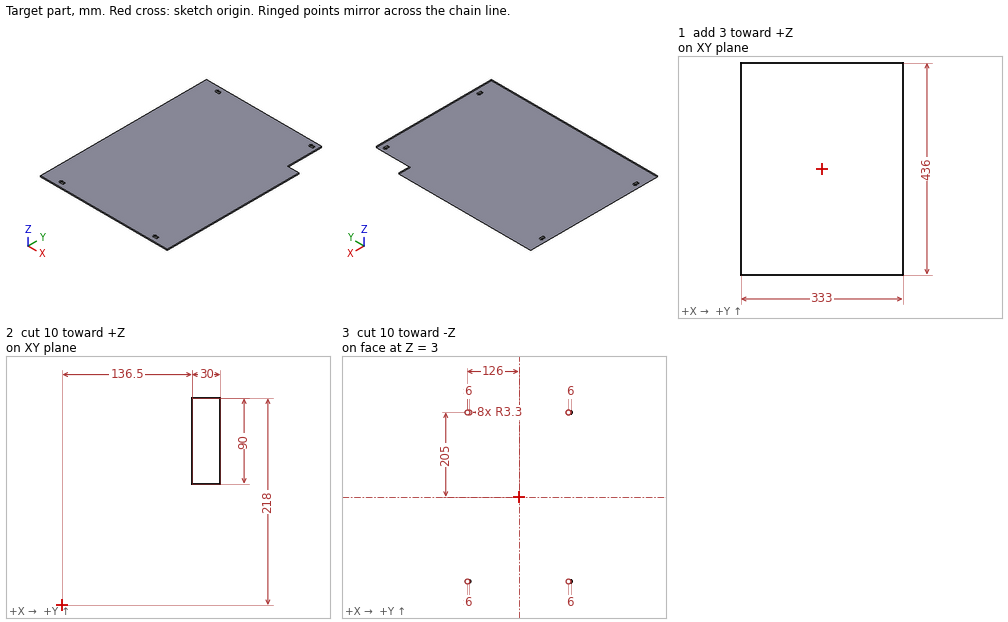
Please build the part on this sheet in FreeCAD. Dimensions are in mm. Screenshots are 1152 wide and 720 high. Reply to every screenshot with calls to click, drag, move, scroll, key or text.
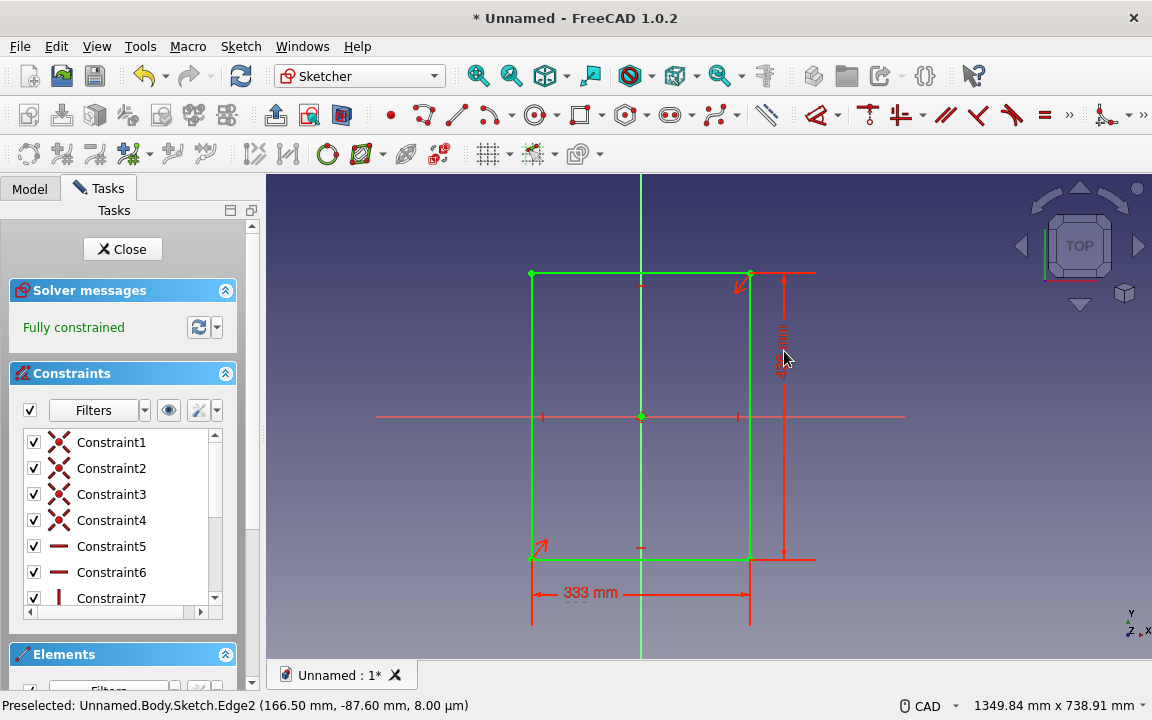
click(123, 249)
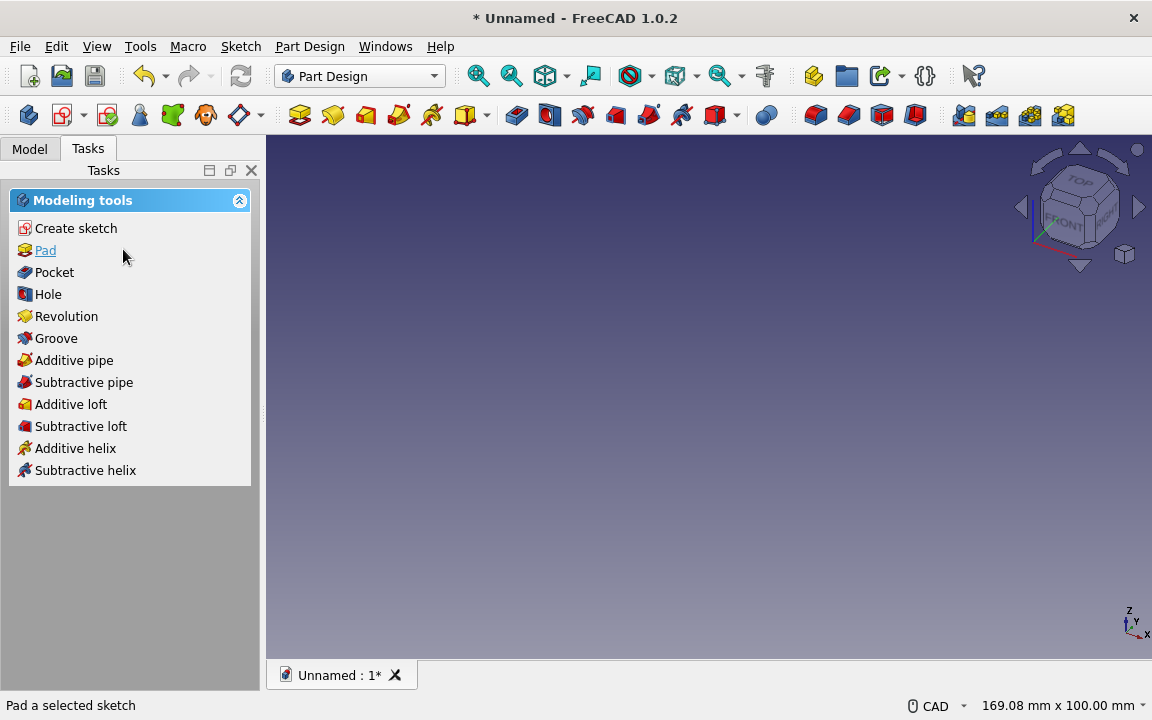
click(300, 116)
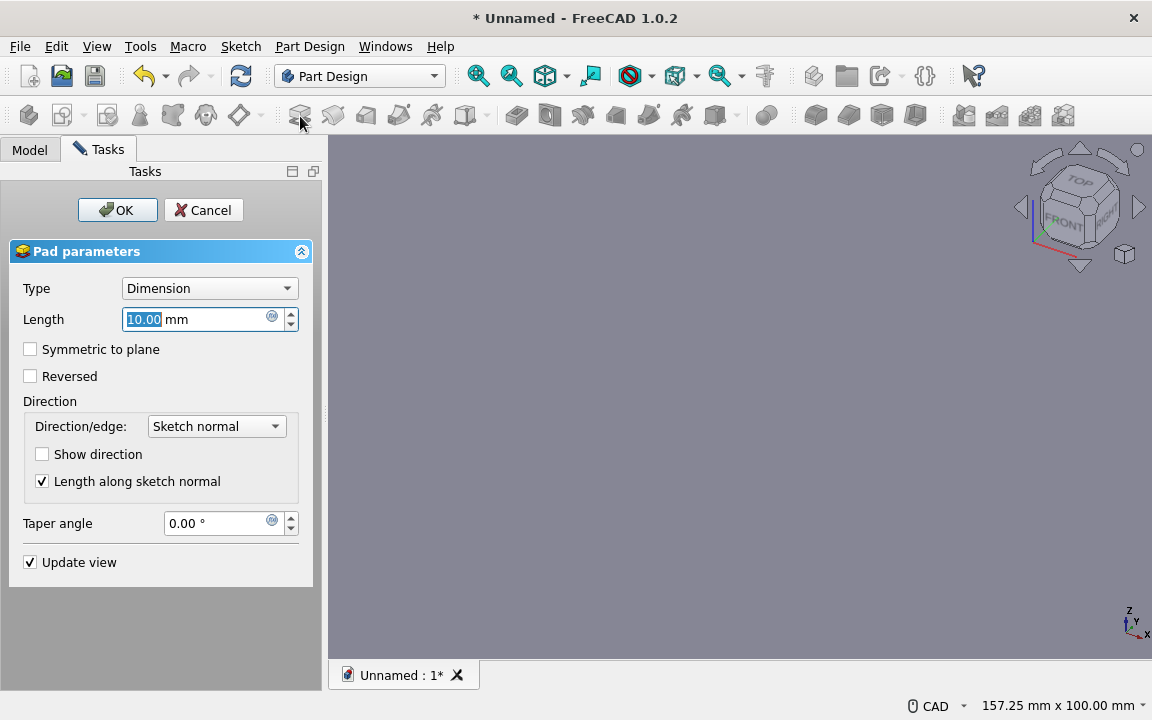
text(3)
key(Tab)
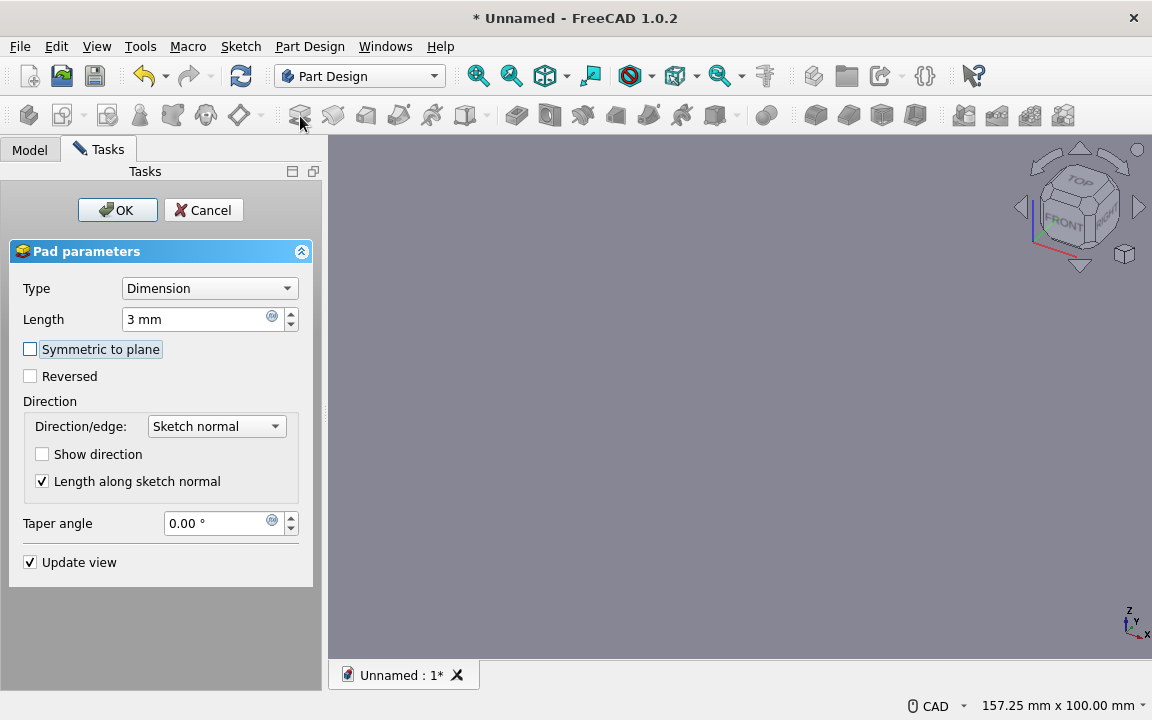
click(118, 210)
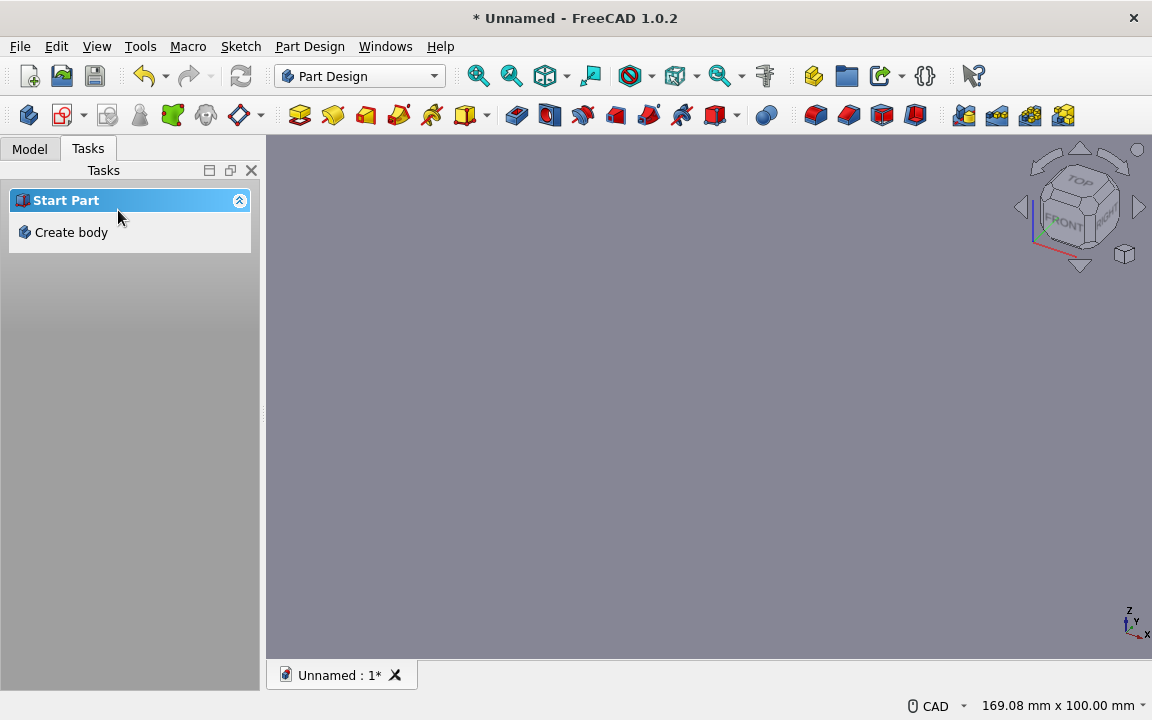
key(v)
key(f)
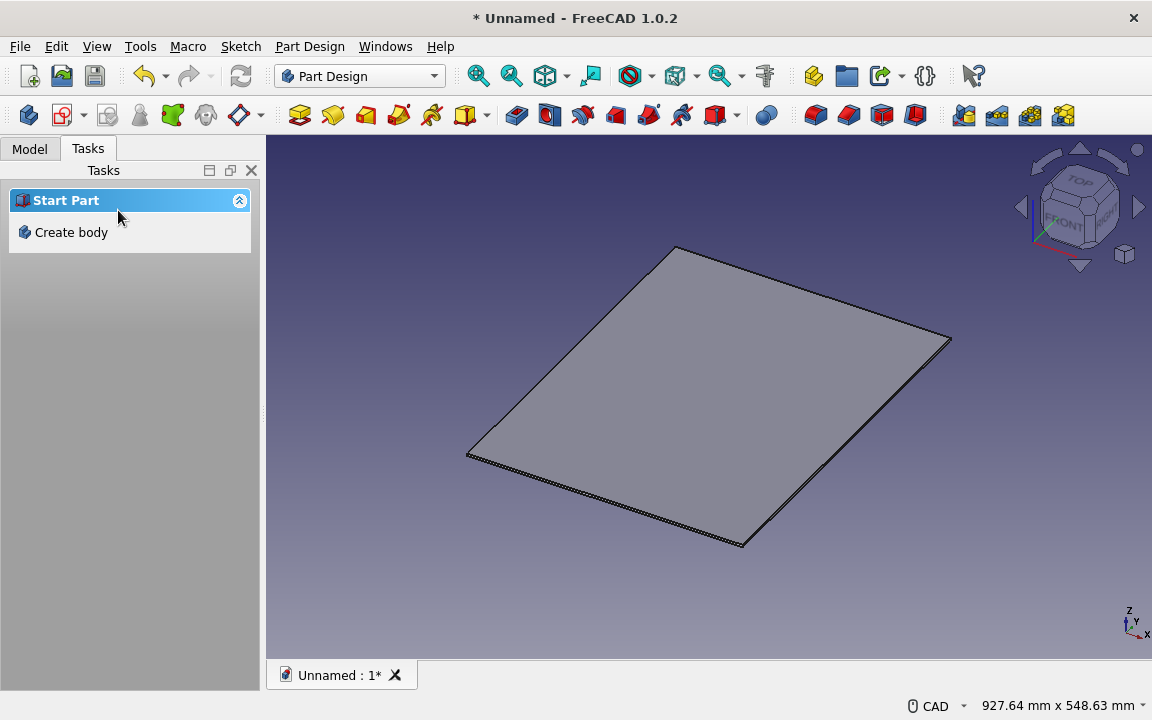
click(62, 116)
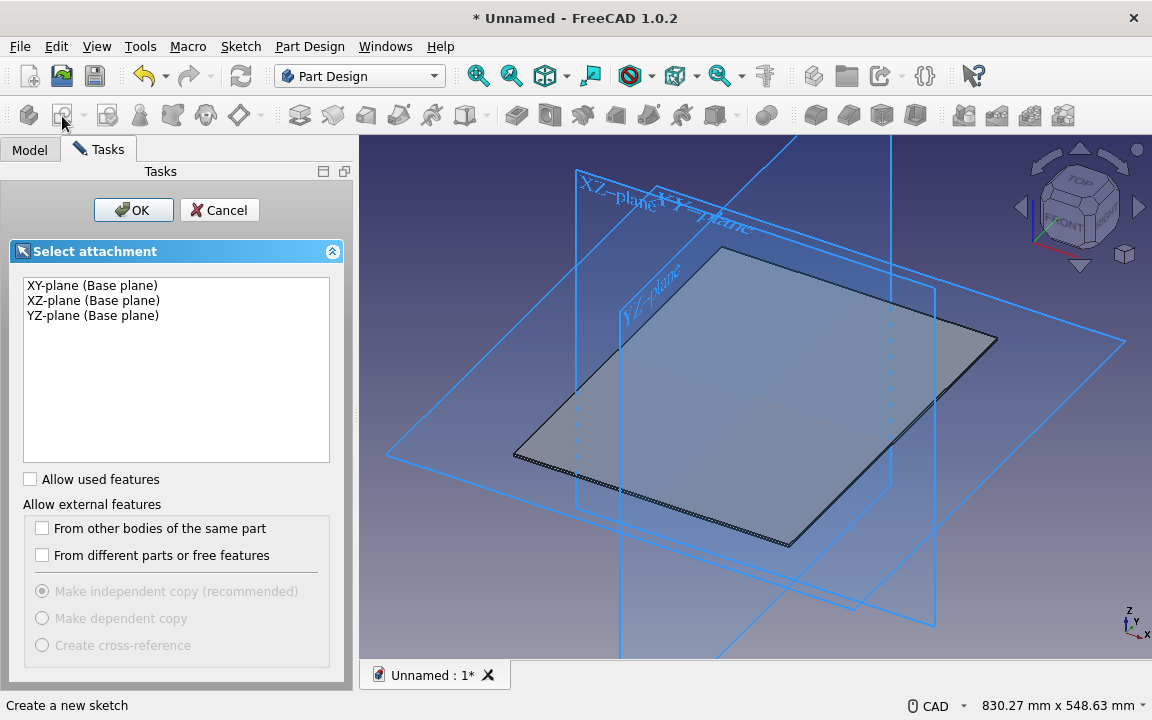
click(84, 286)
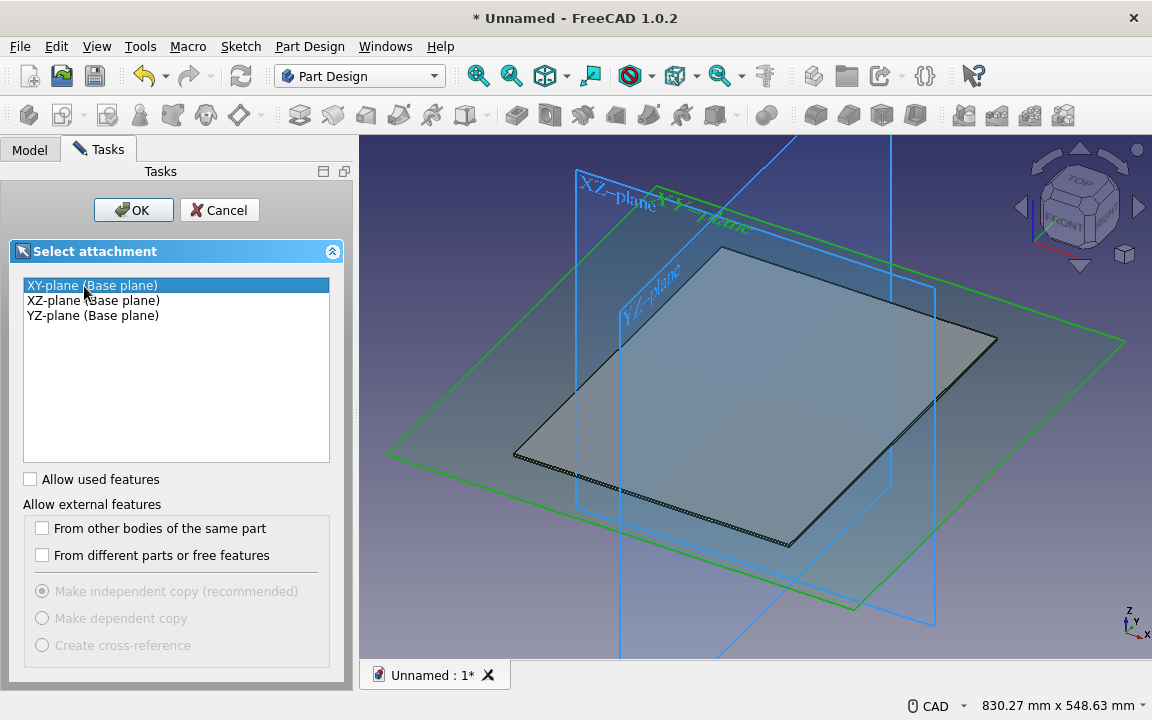
click(134, 210)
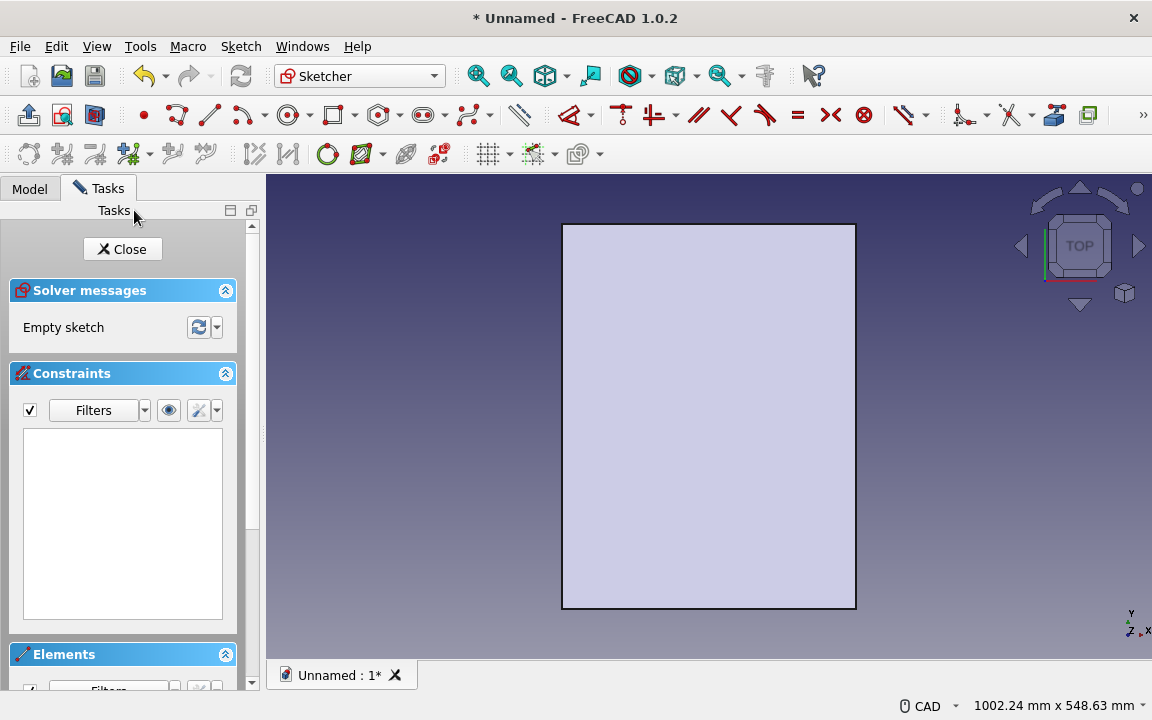
click(95, 116)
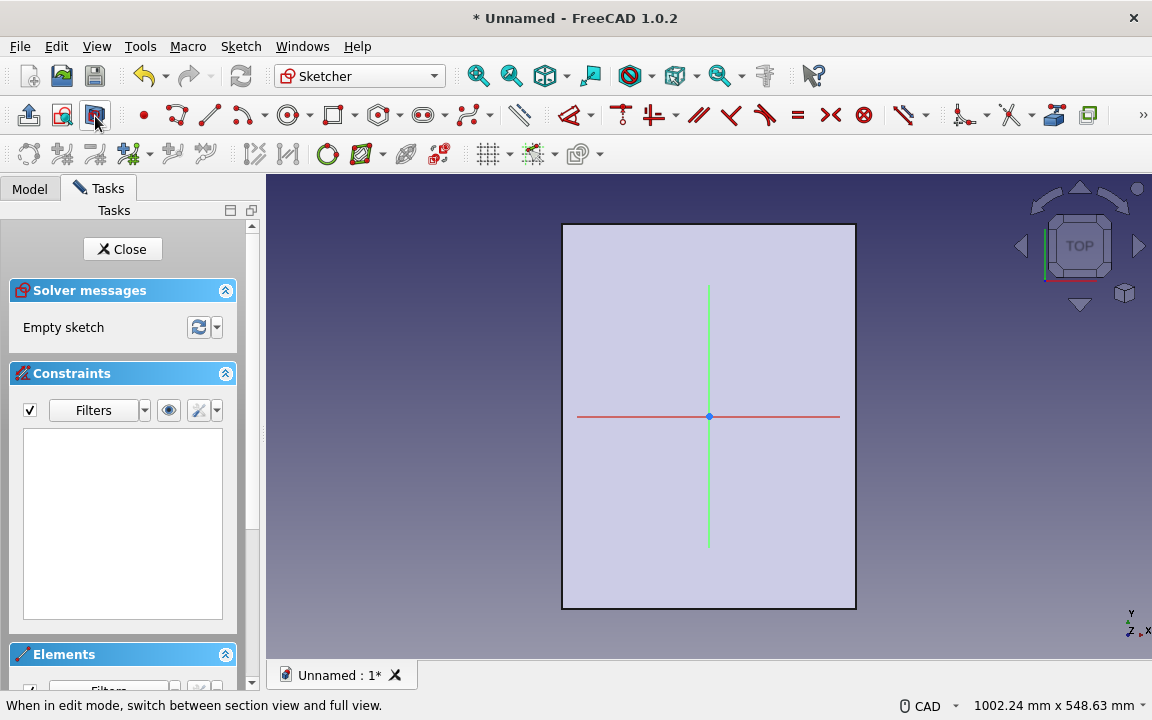
scroll(987, 202, up, 2)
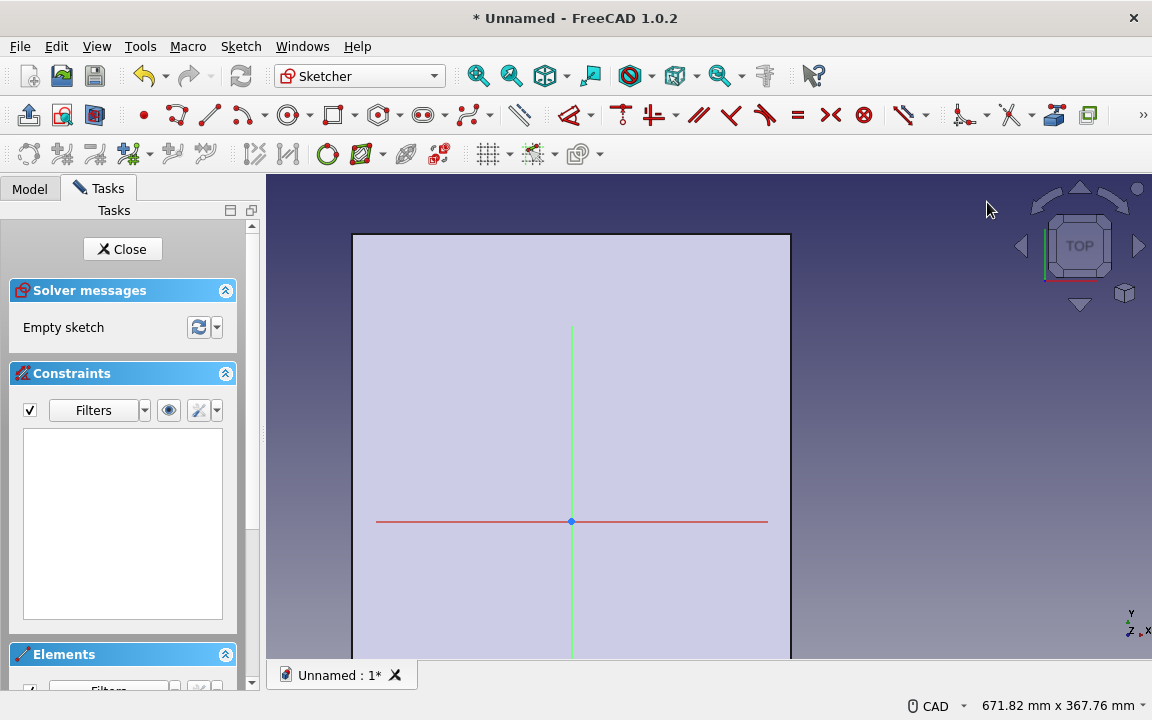
click(332, 116)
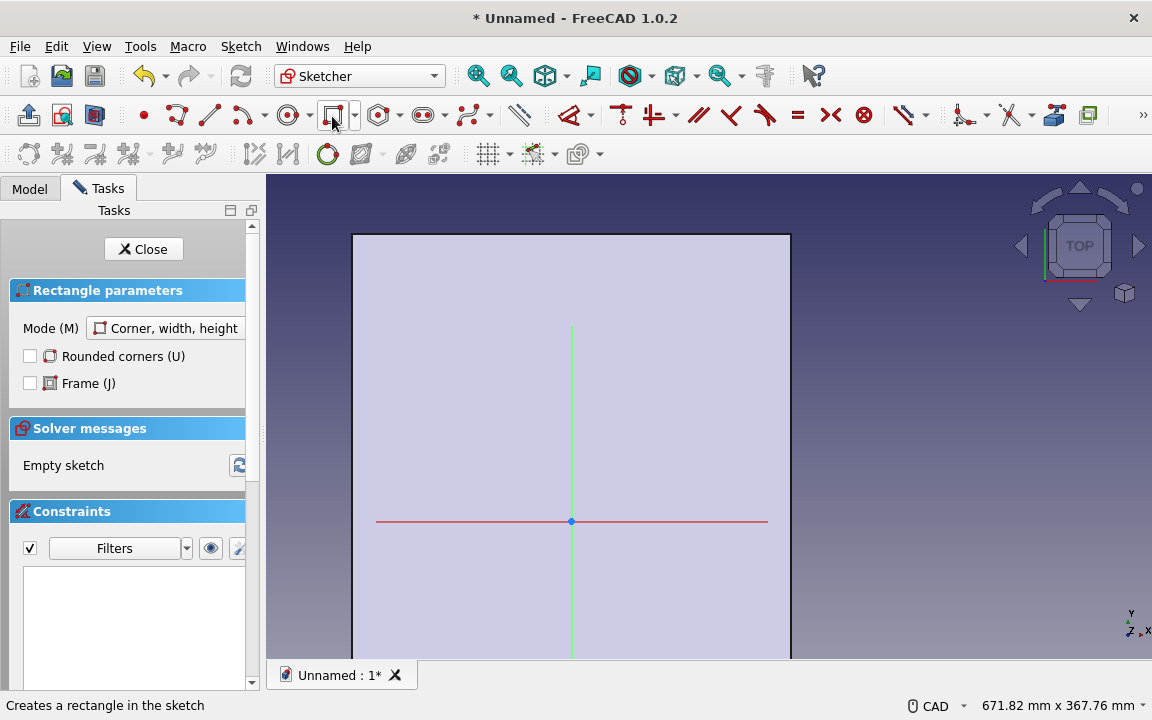
click(752, 234)
click(791, 353)
key(Escape)